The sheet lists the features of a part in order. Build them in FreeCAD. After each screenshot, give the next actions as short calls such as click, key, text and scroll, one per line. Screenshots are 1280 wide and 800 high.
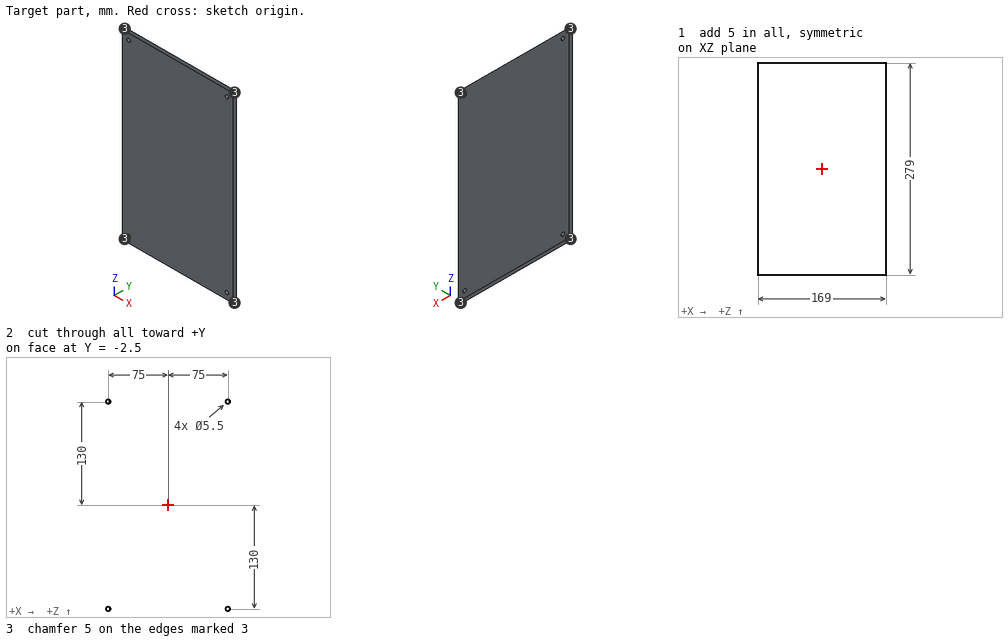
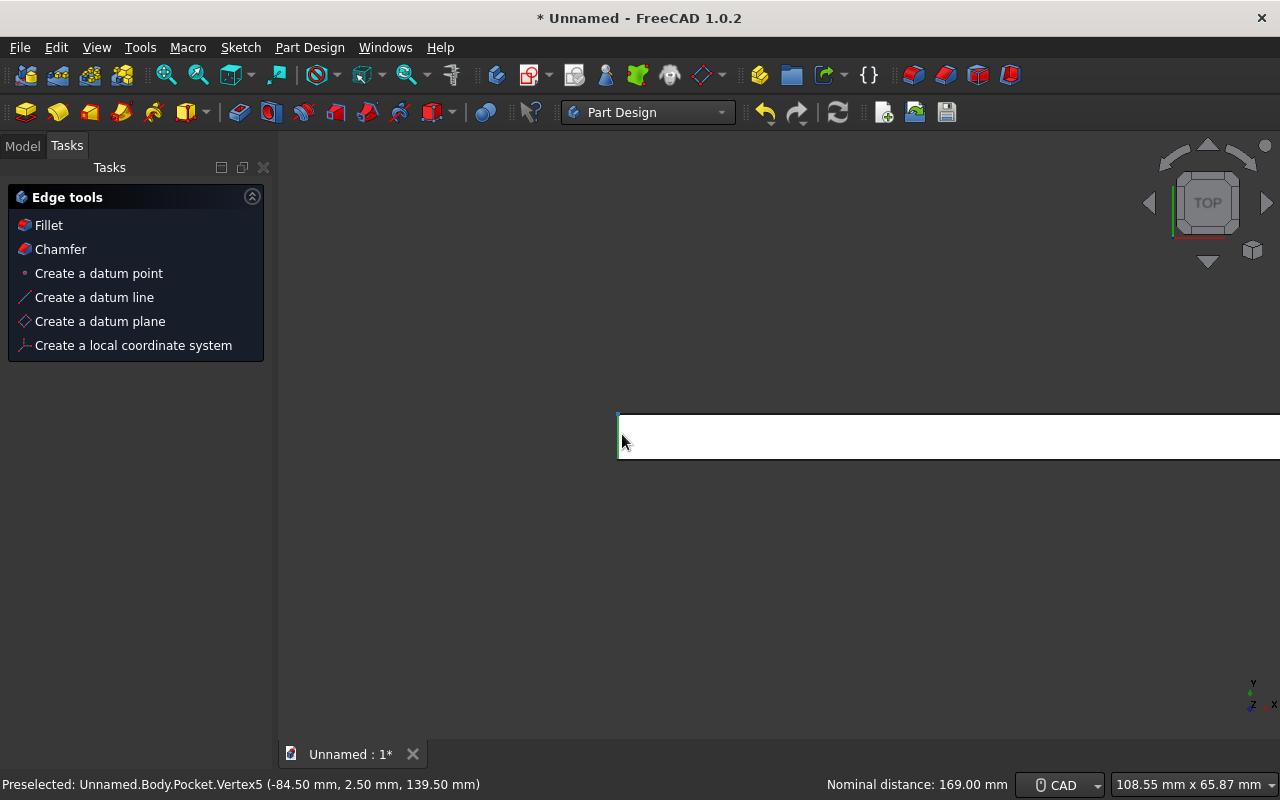
click(168, 76)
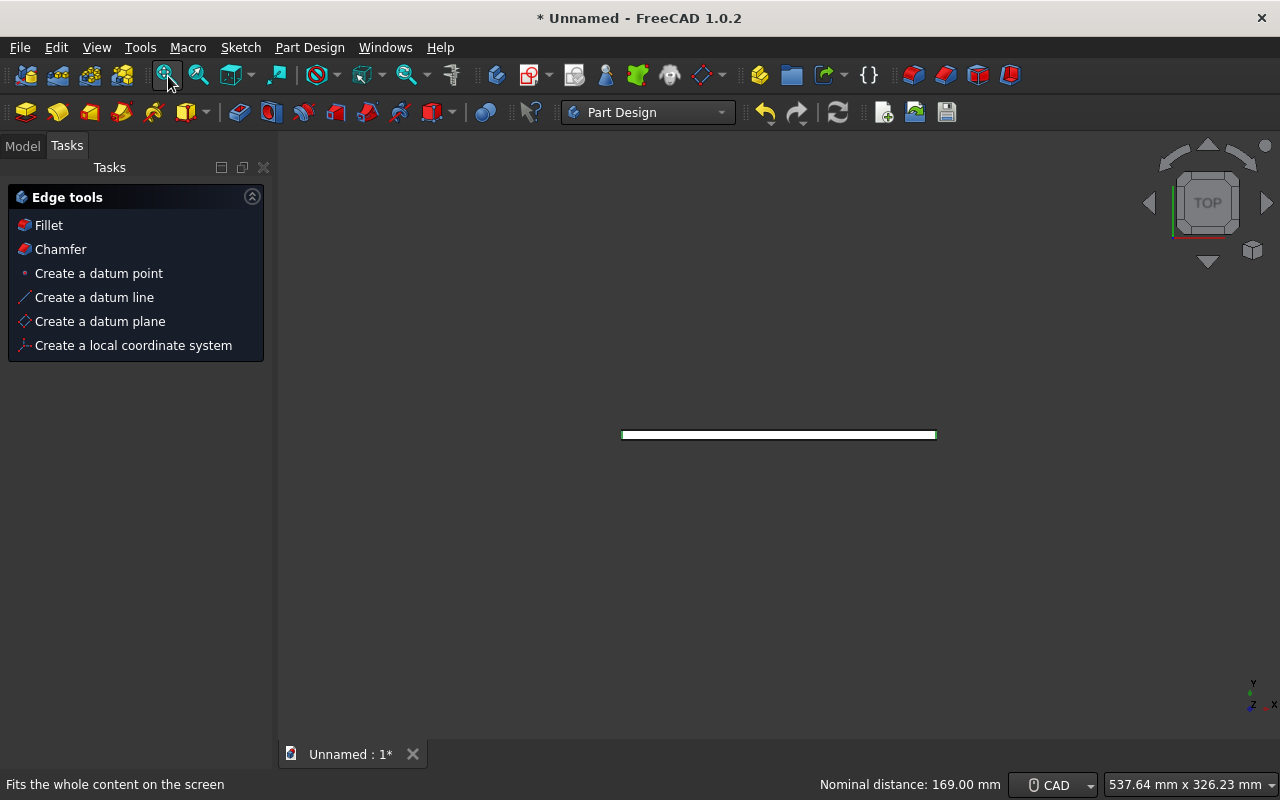
key(1)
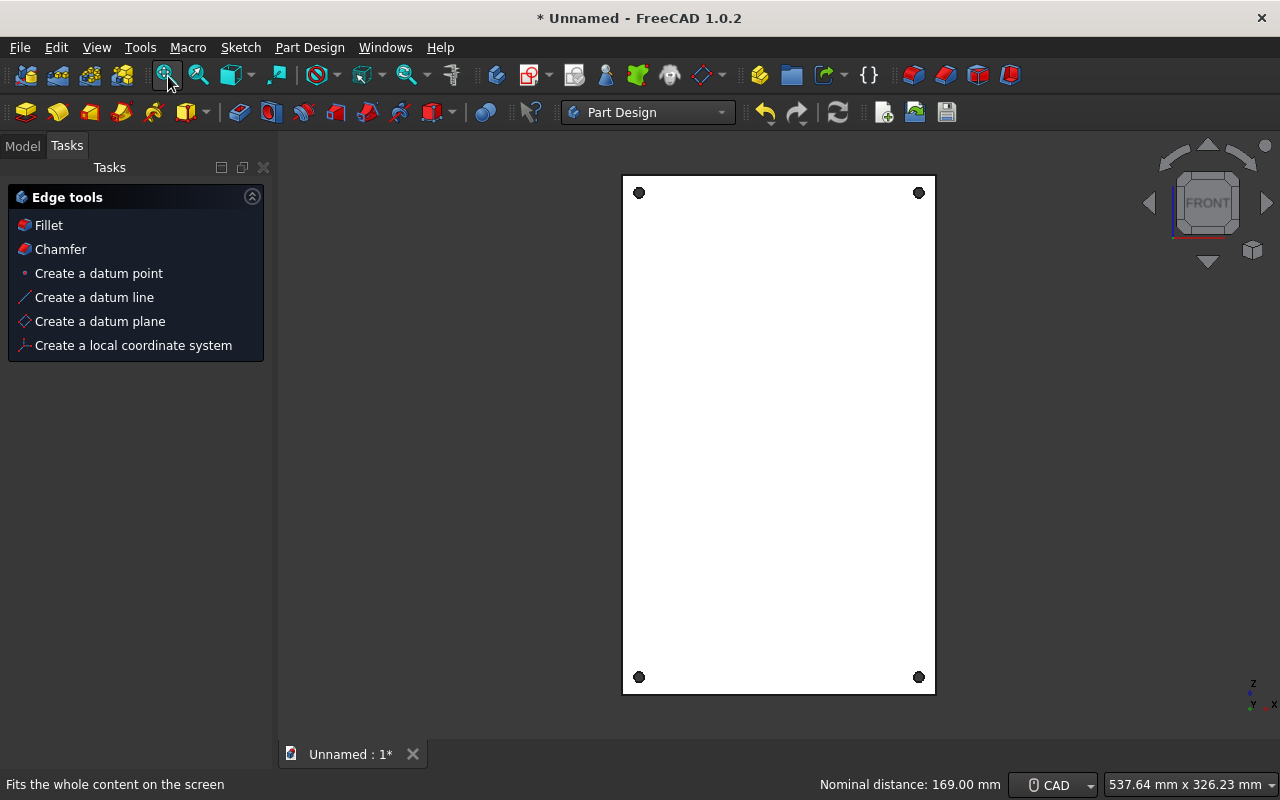
scroll(622, 694, up, 8)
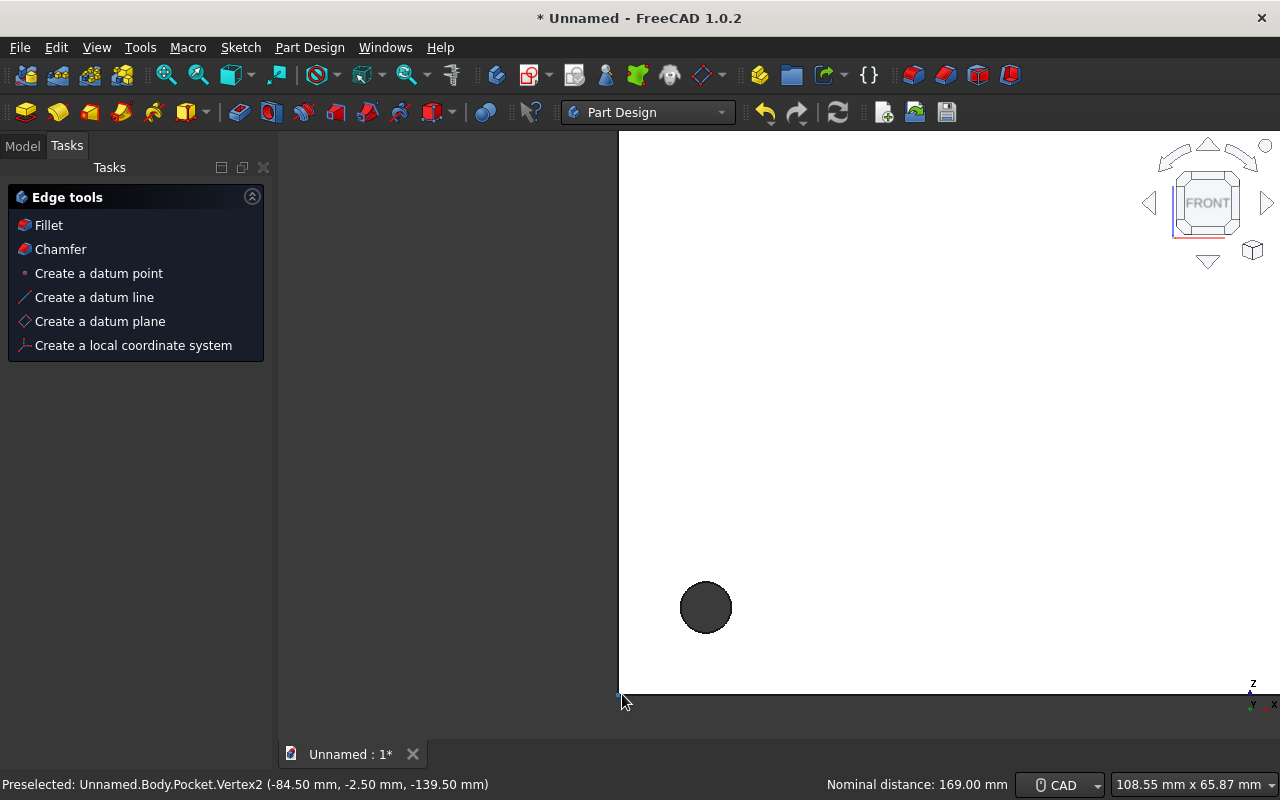
click(168, 76)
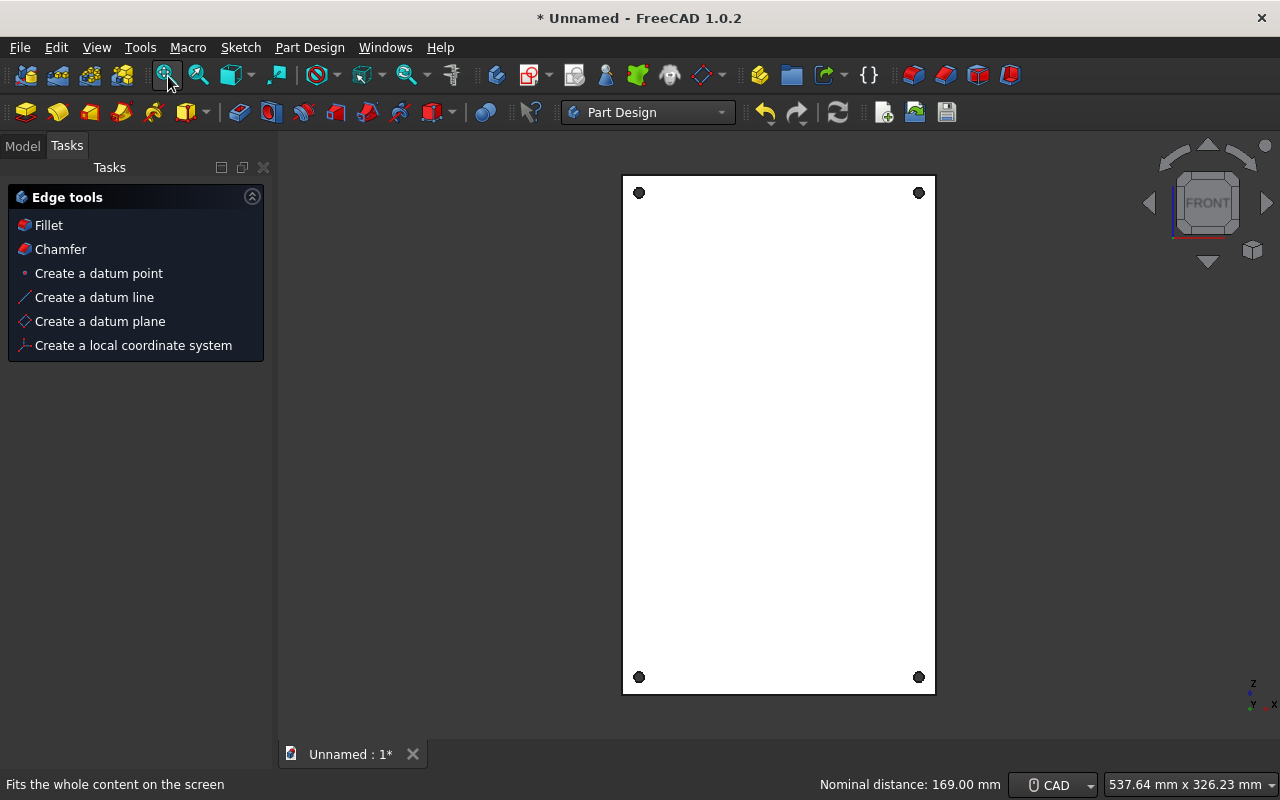
key(3)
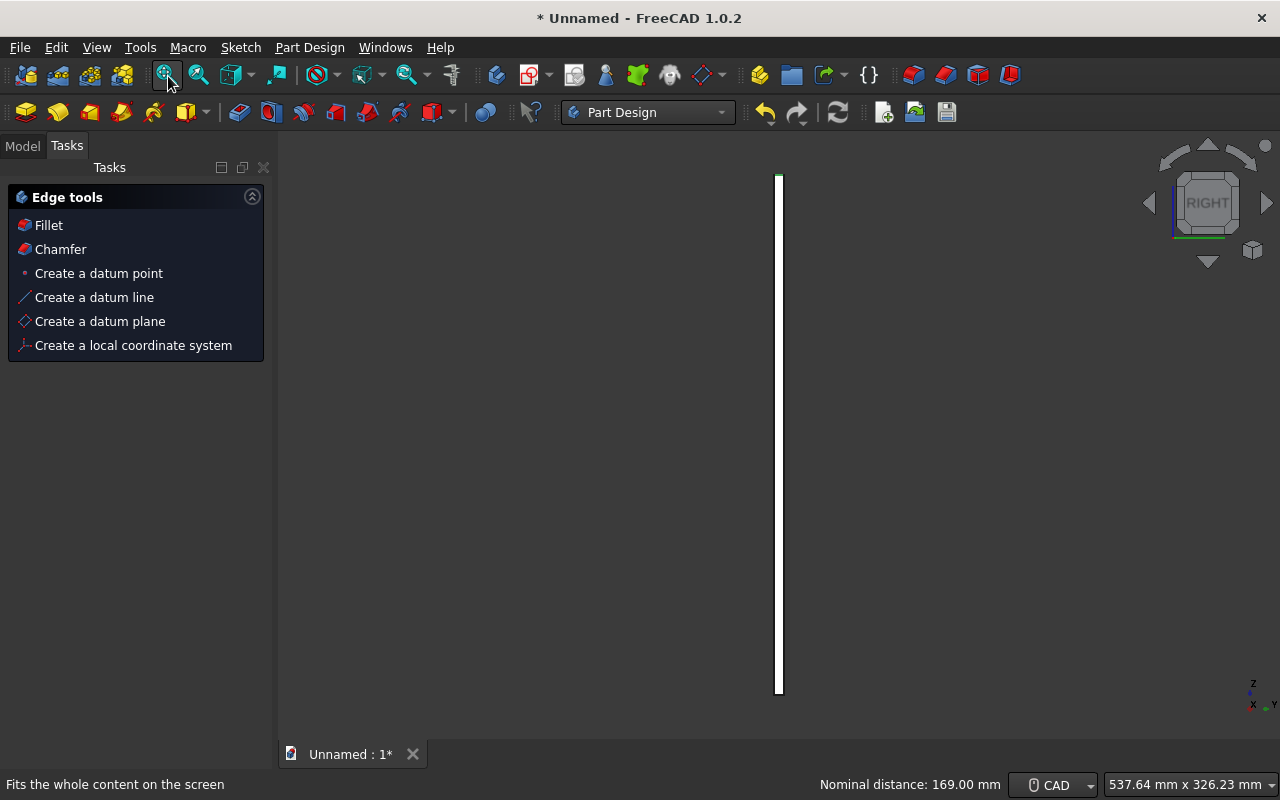
scroll(779, 694, up, 8)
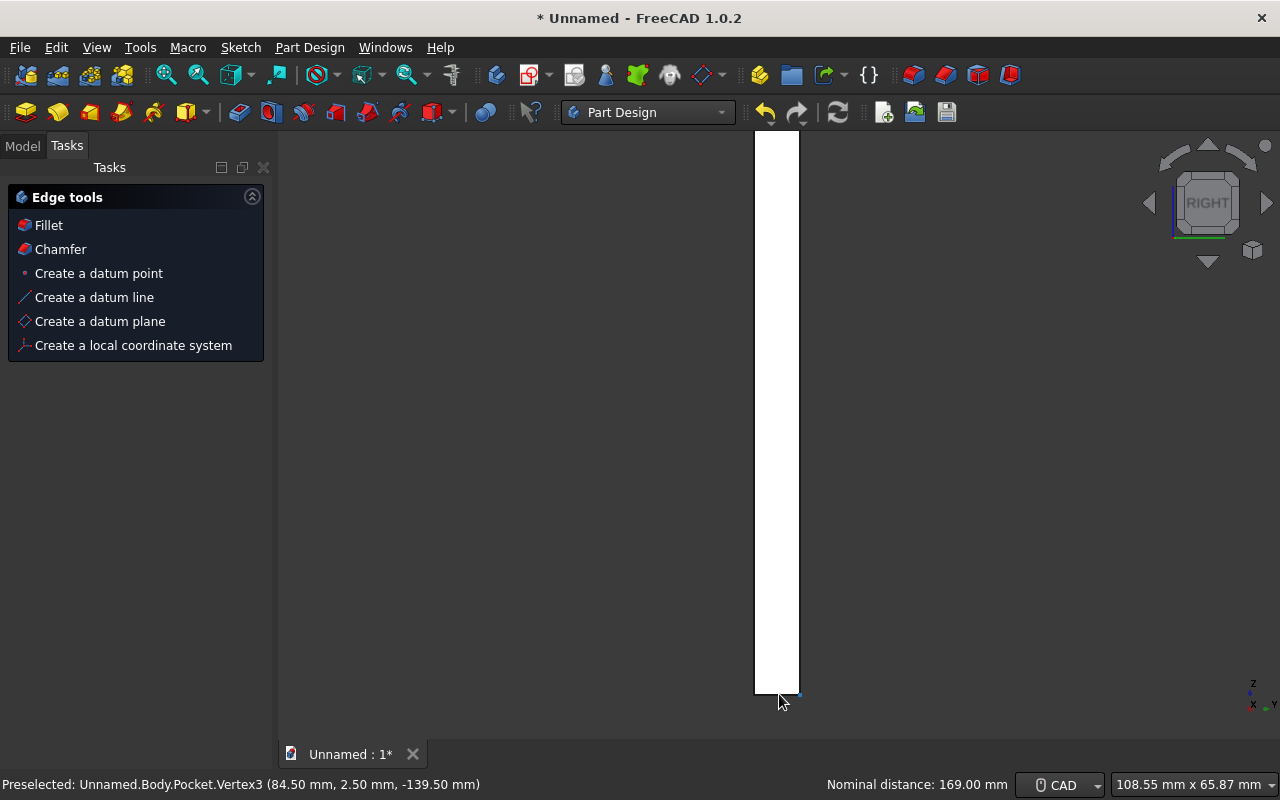
click(777, 694, ctrl)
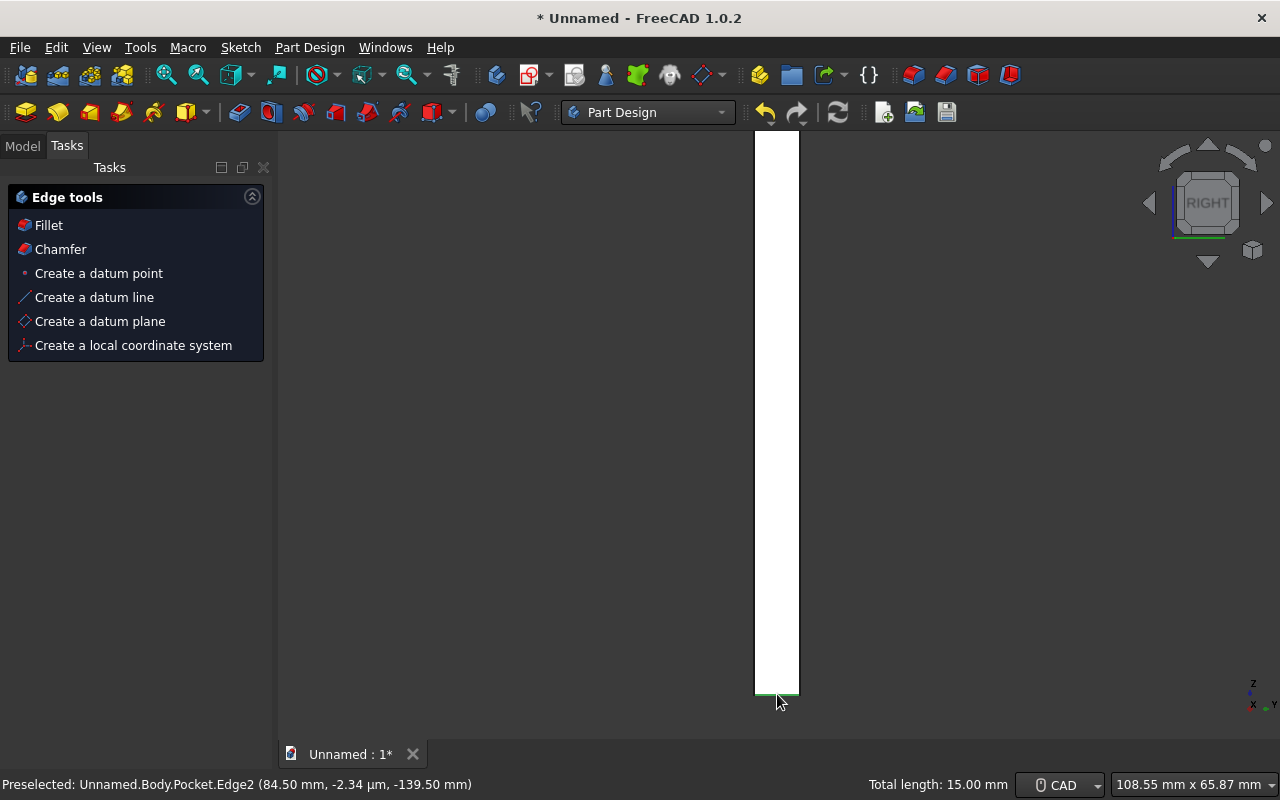
click(168, 76)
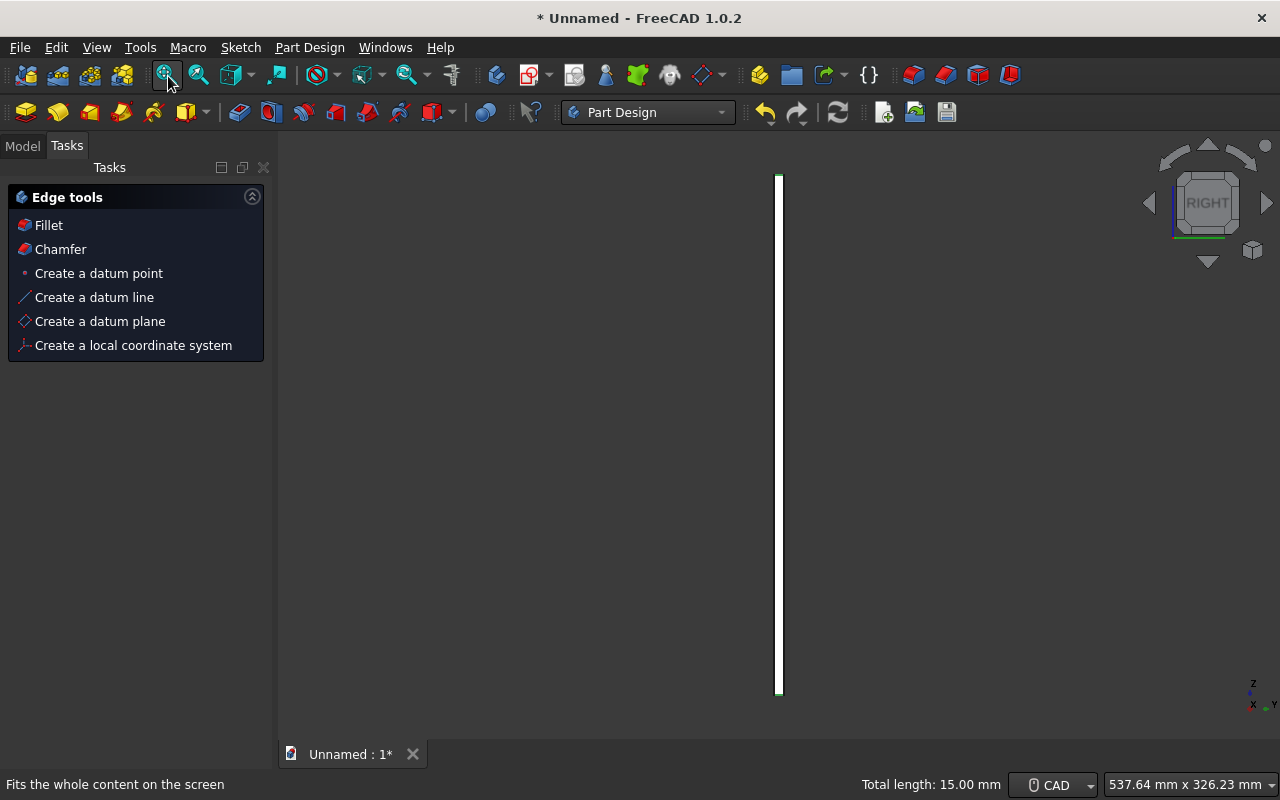
key(5)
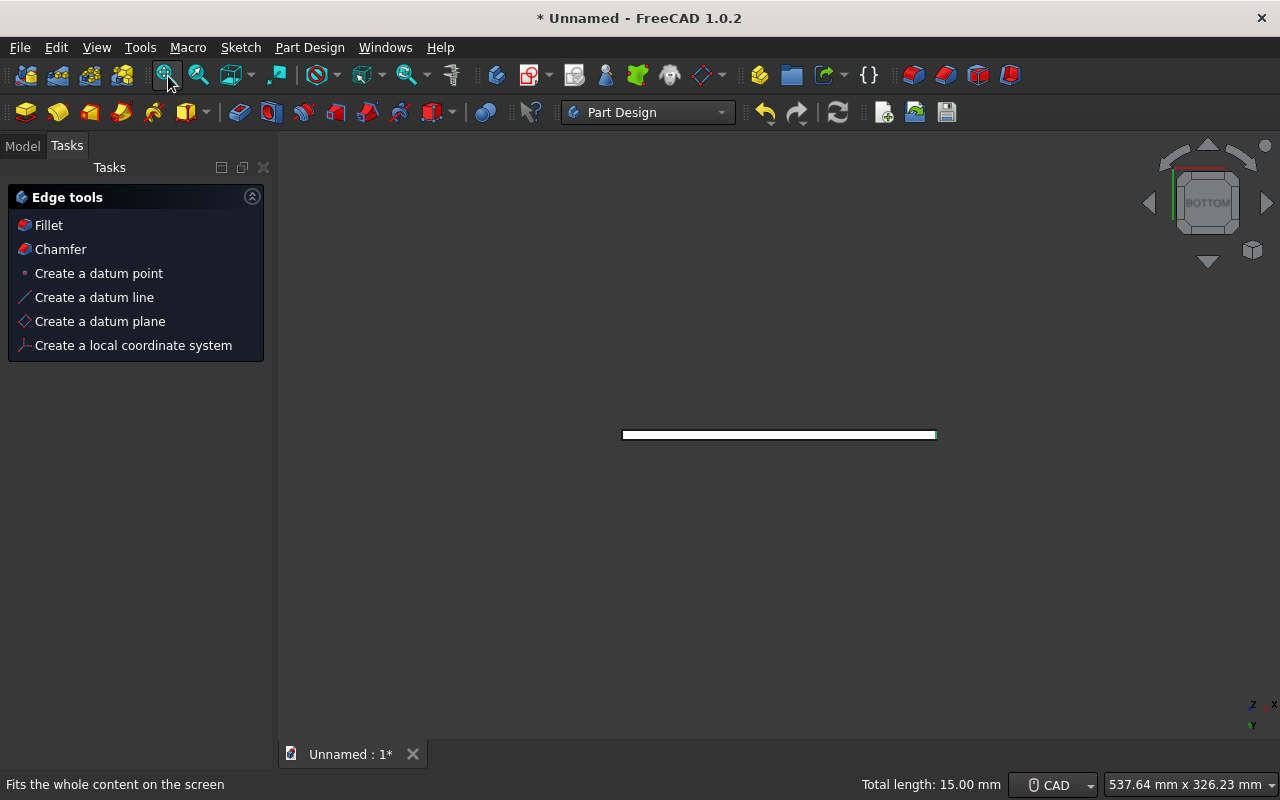
click(168, 76)